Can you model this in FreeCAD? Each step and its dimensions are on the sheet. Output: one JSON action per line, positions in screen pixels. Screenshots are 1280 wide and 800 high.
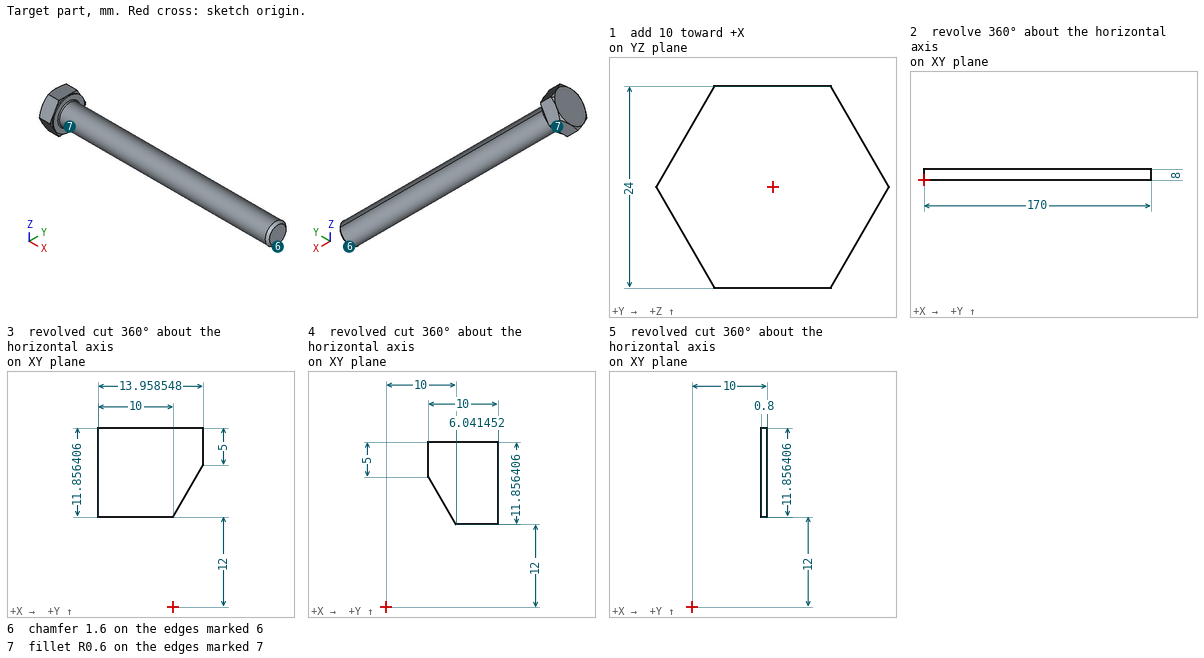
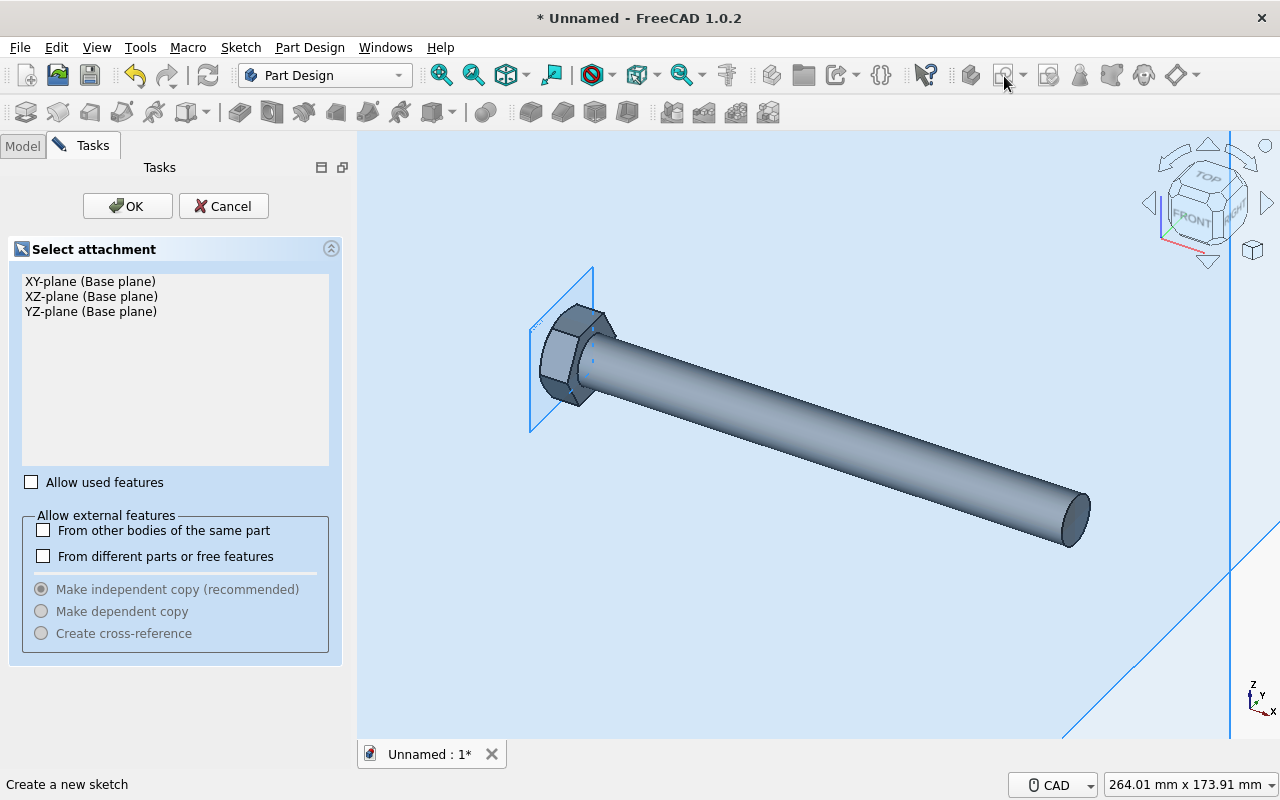
{"action": "left_click", "coordinate": [82, 282]}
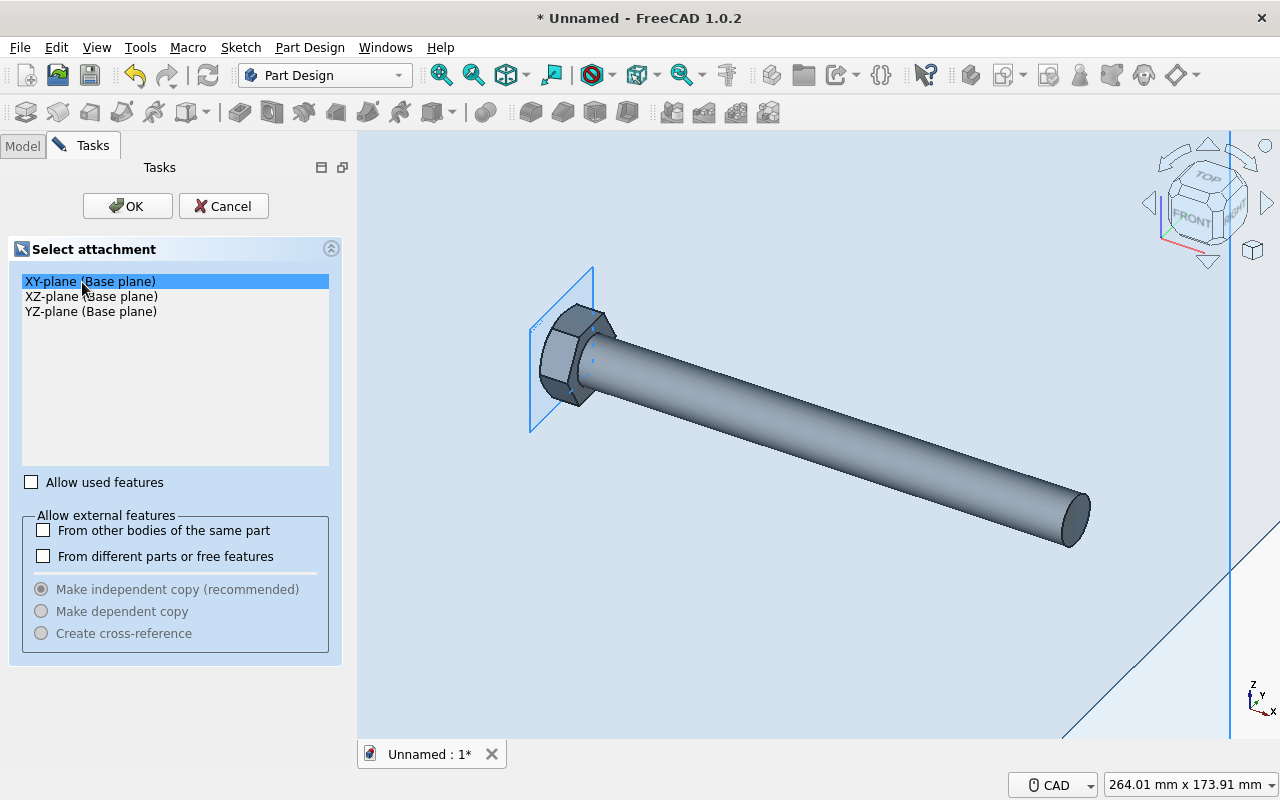
{"action": "left_click", "coordinate": [128, 206]}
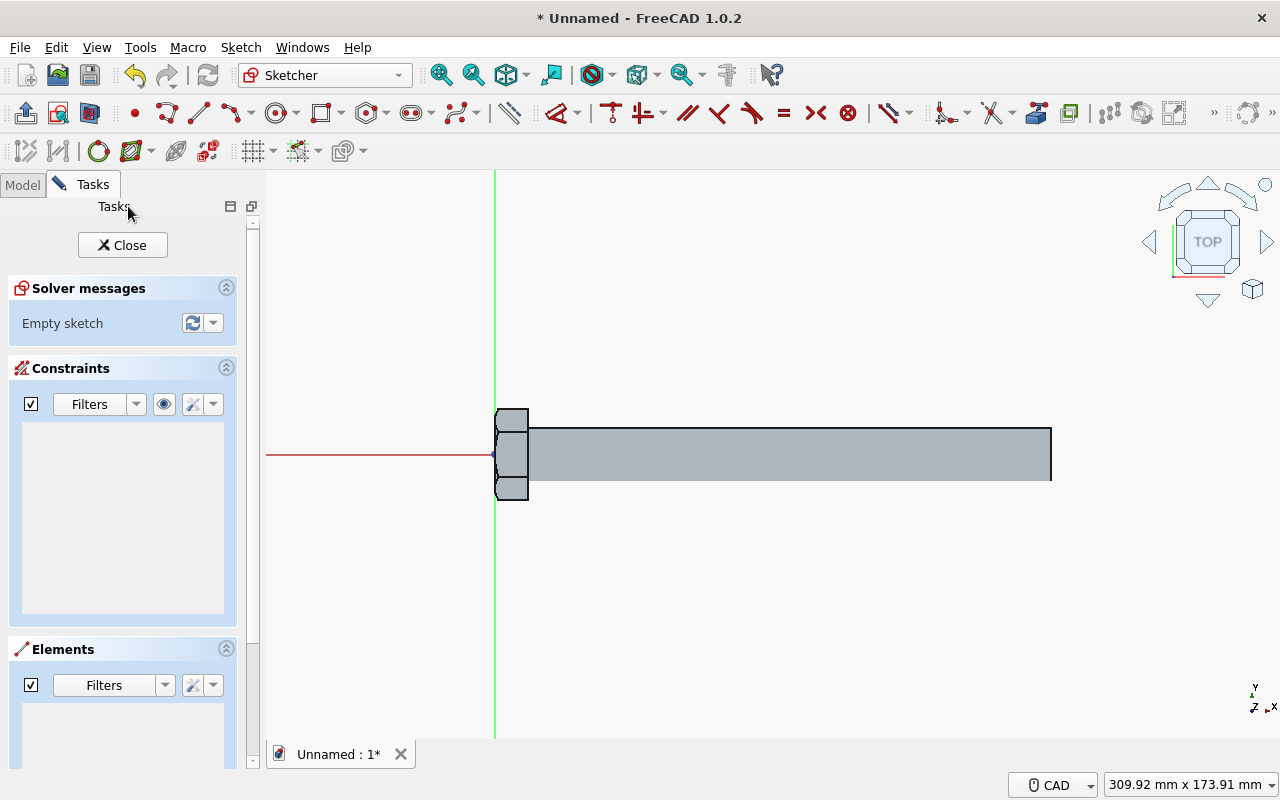
{"action": "left_click", "coordinate": [90, 114]}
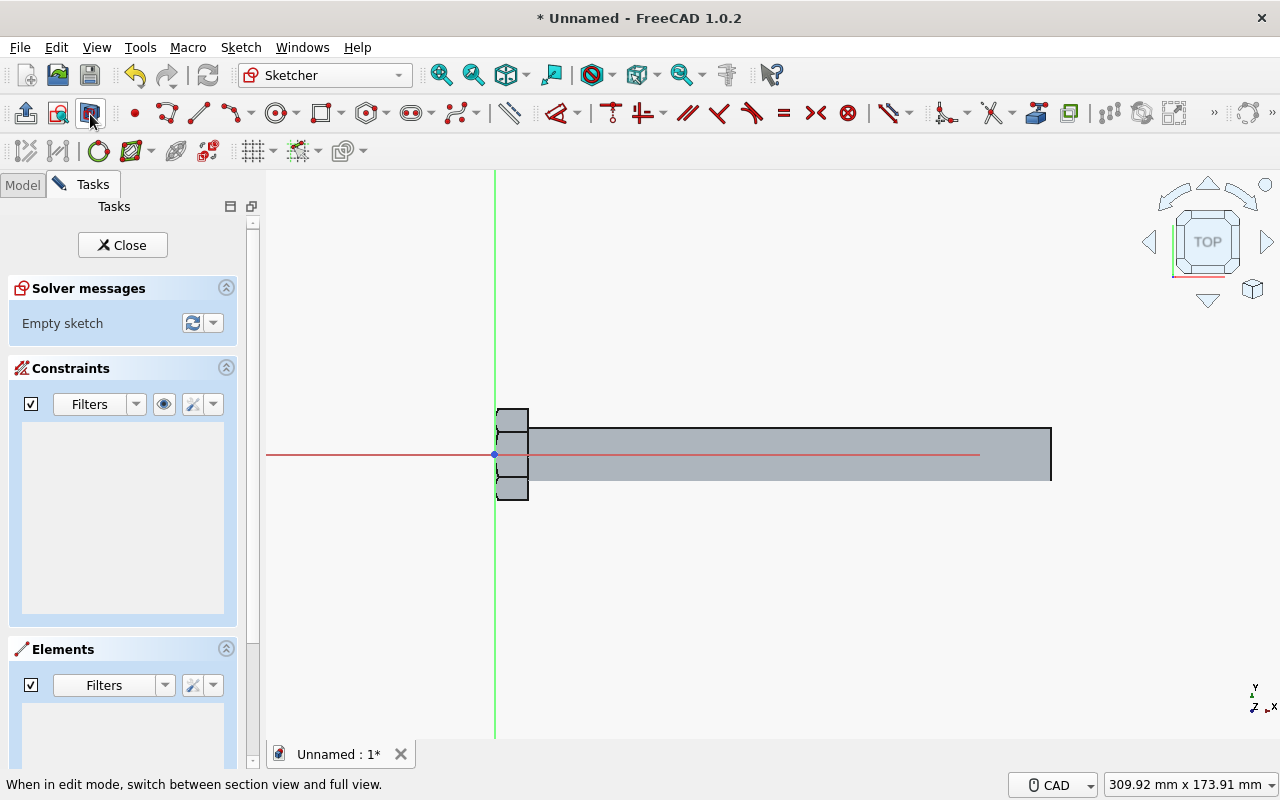
{"action": "scroll", "coordinate": [475, 406], "scroll_direction": "up", "scroll_amount": 8}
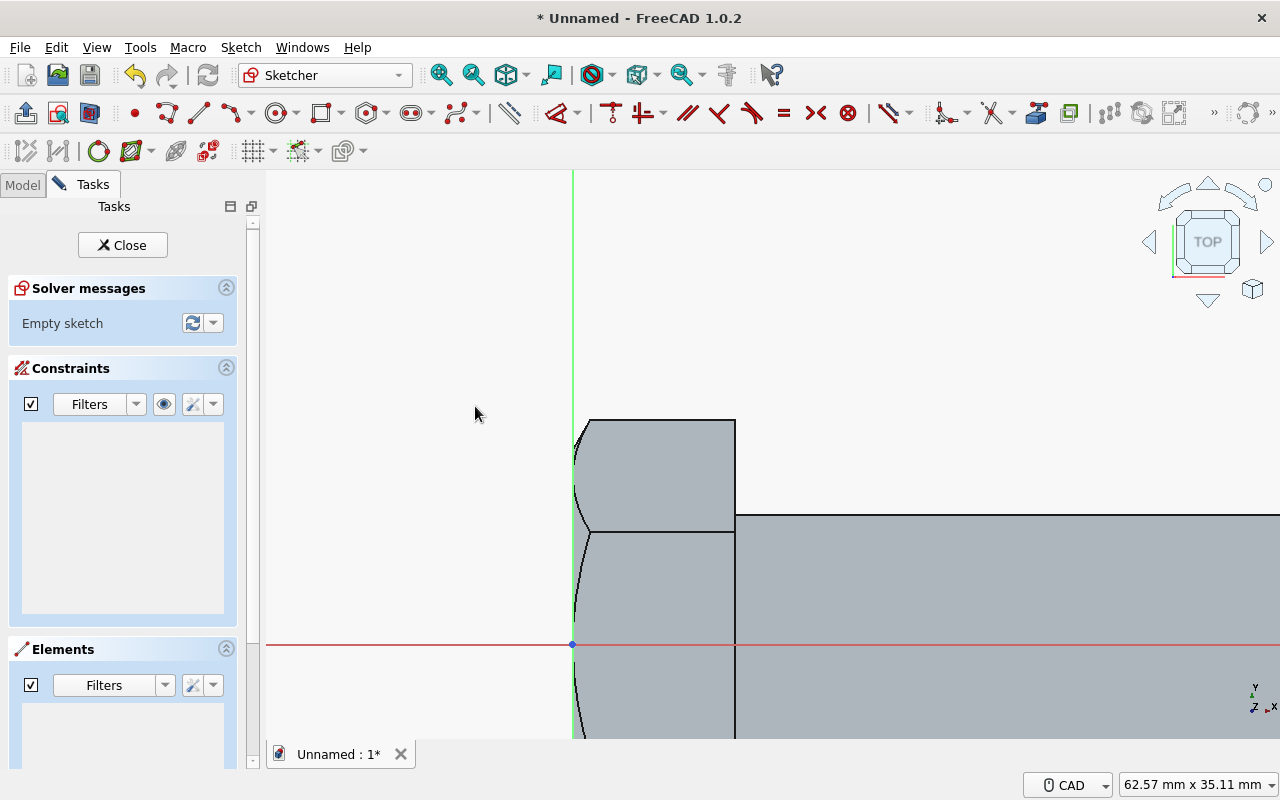
{"action": "left_click", "coordinate": [168, 114]}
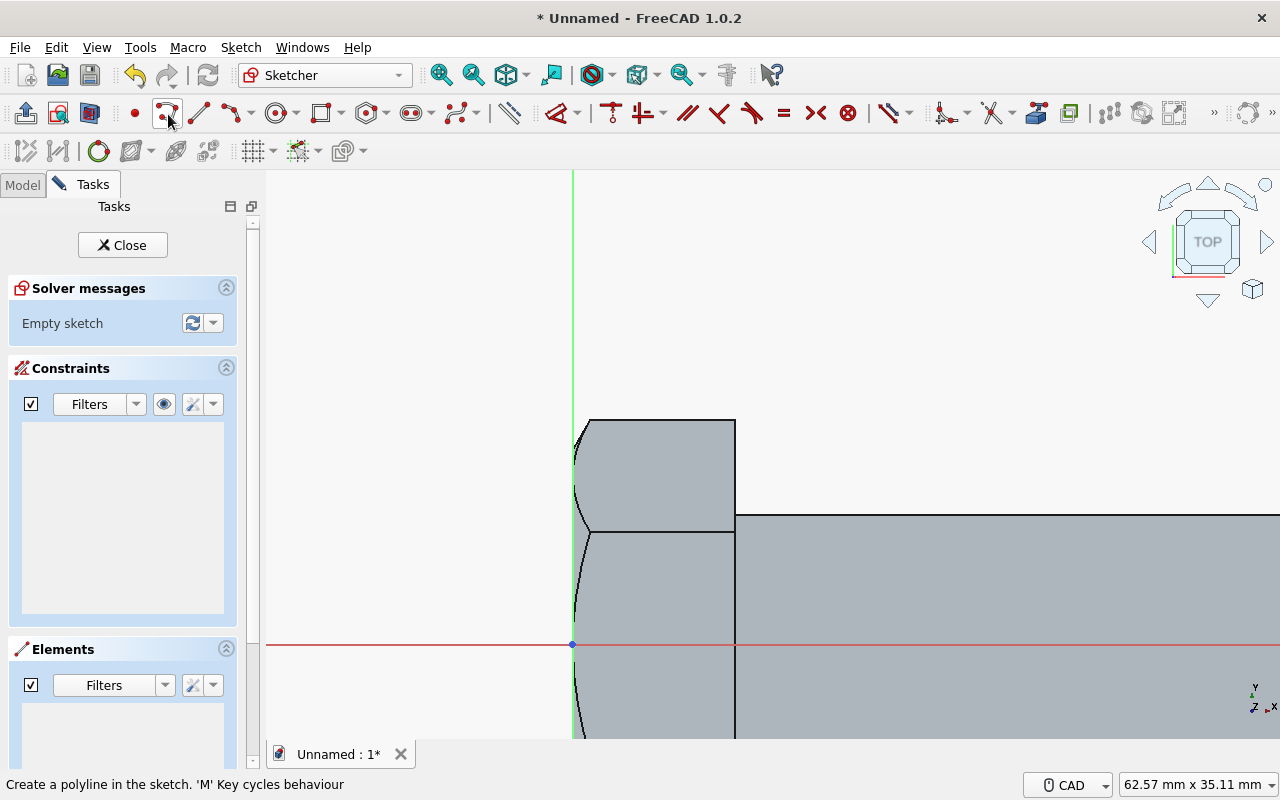
{"action": "left_click", "coordinate": [735, 450]}
{"action": "left_click", "coordinate": [833, 450]}
{"action": "left_click", "coordinate": [833, 258]}
{"action": "left_click", "coordinate": [671, 258]}
{"action": "left_click", "coordinate": [671, 339]}
{"action": "left_click", "coordinate": [735, 451]}
{"action": "key", "text": "Escape"}
{"action": "key", "text": "Escape"}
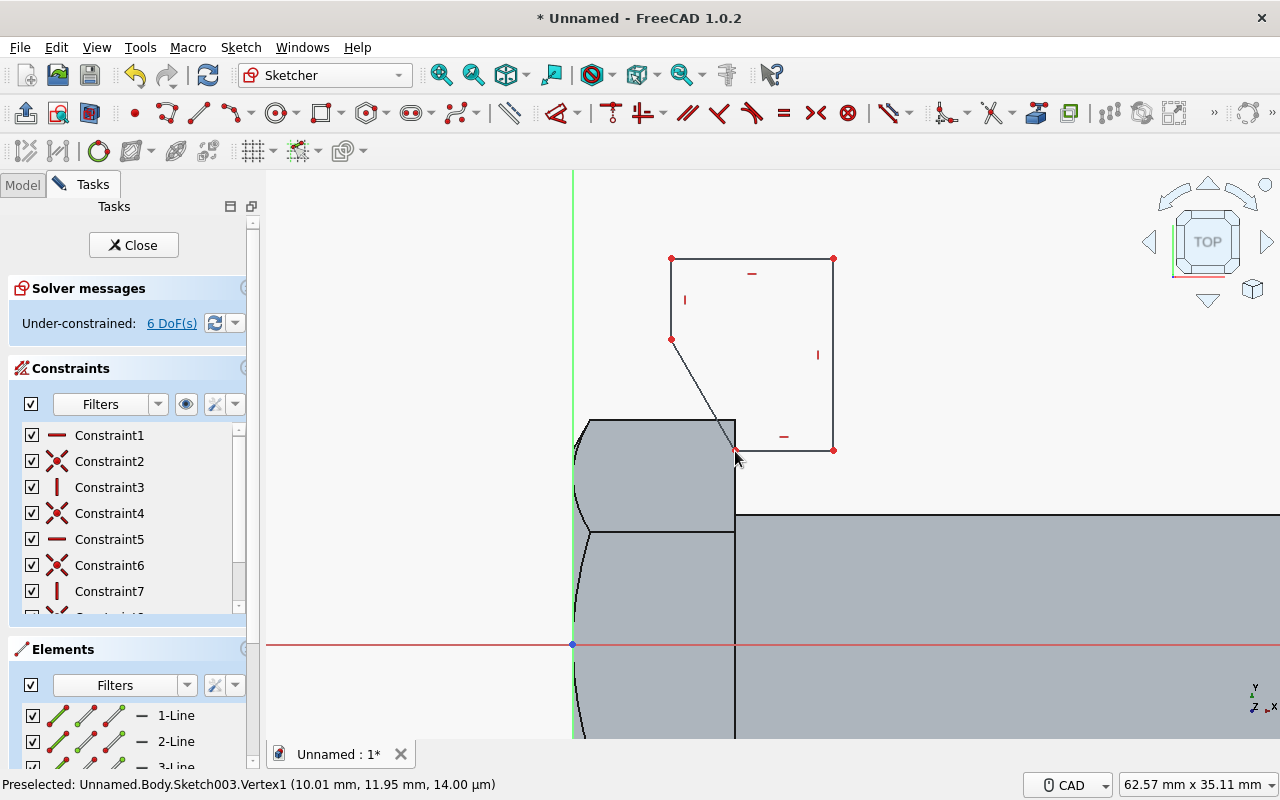
{"action": "left_click", "coordinate": [556, 114]}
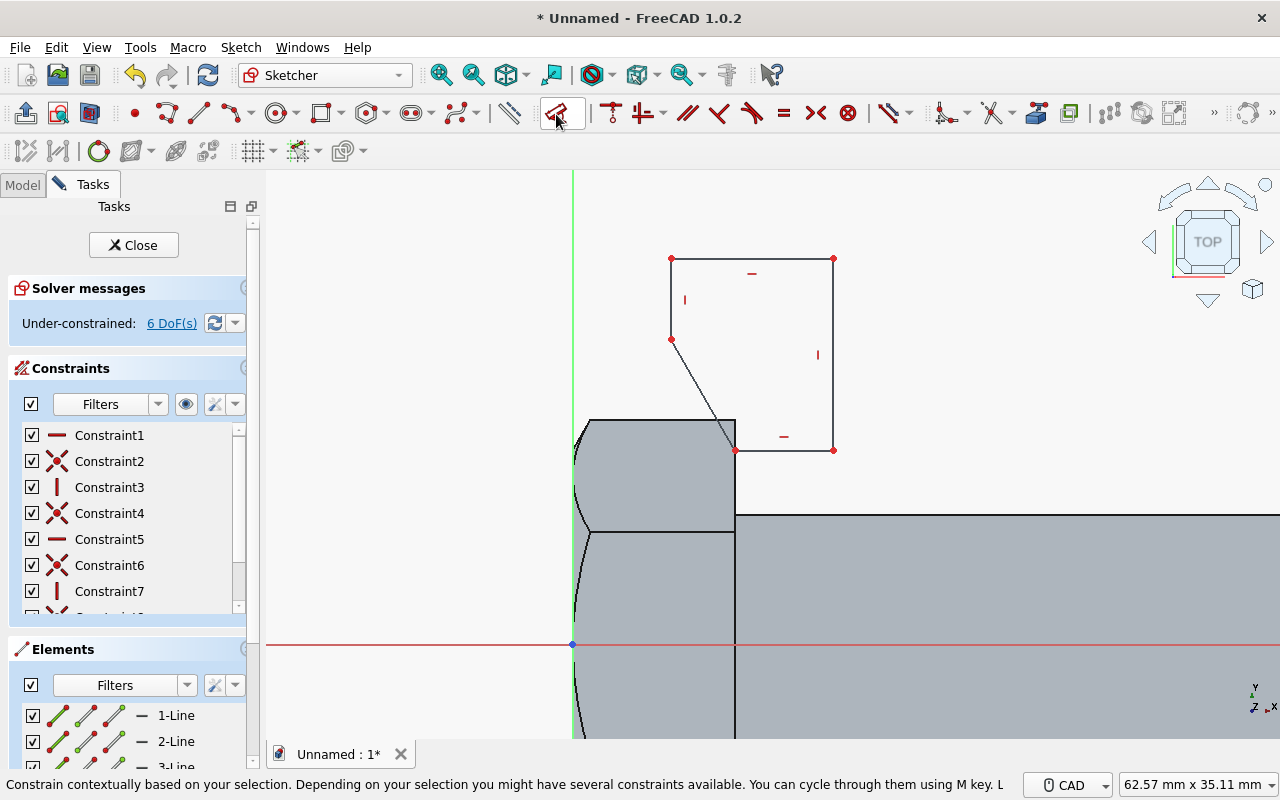
{"action": "left_click", "coordinate": [671, 283]}
{"action": "left_click", "coordinate": [637, 299]}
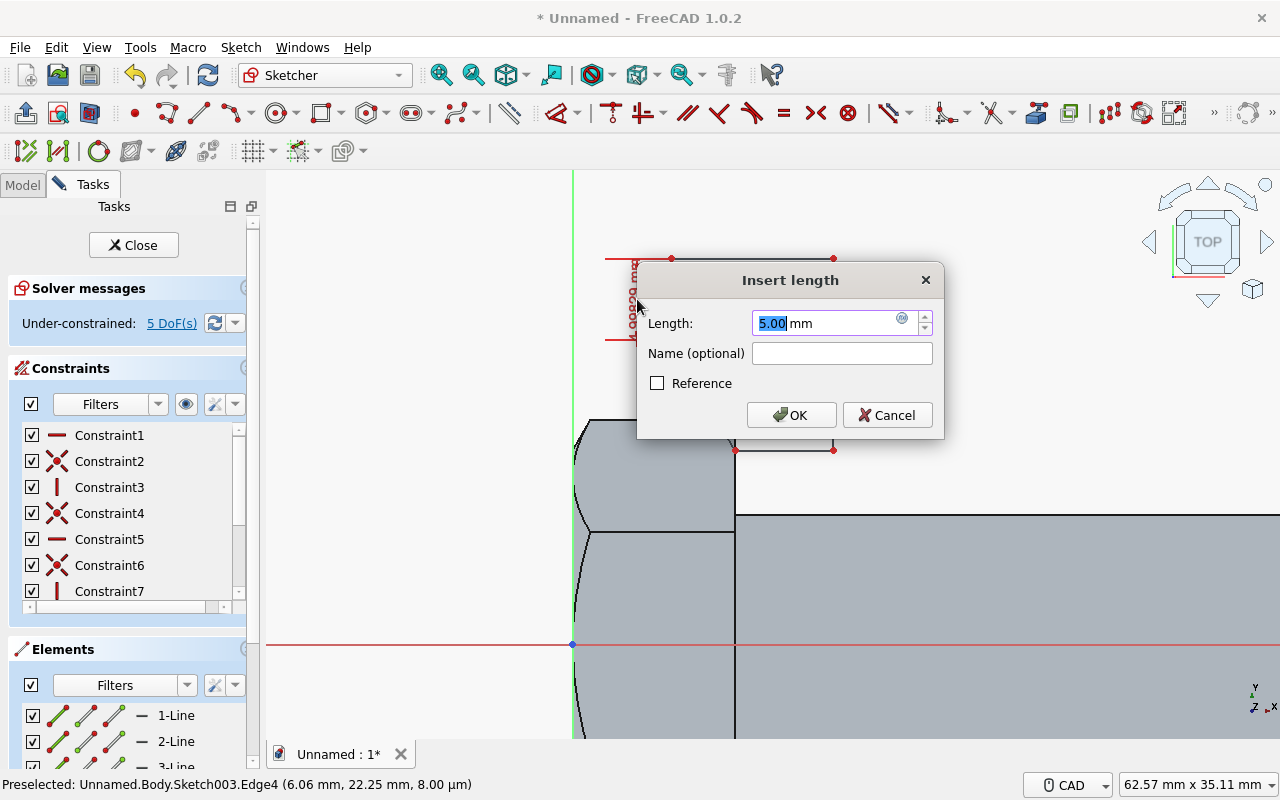
{"action": "type", "text": "5"}
{"action": "key", "text": "Return"}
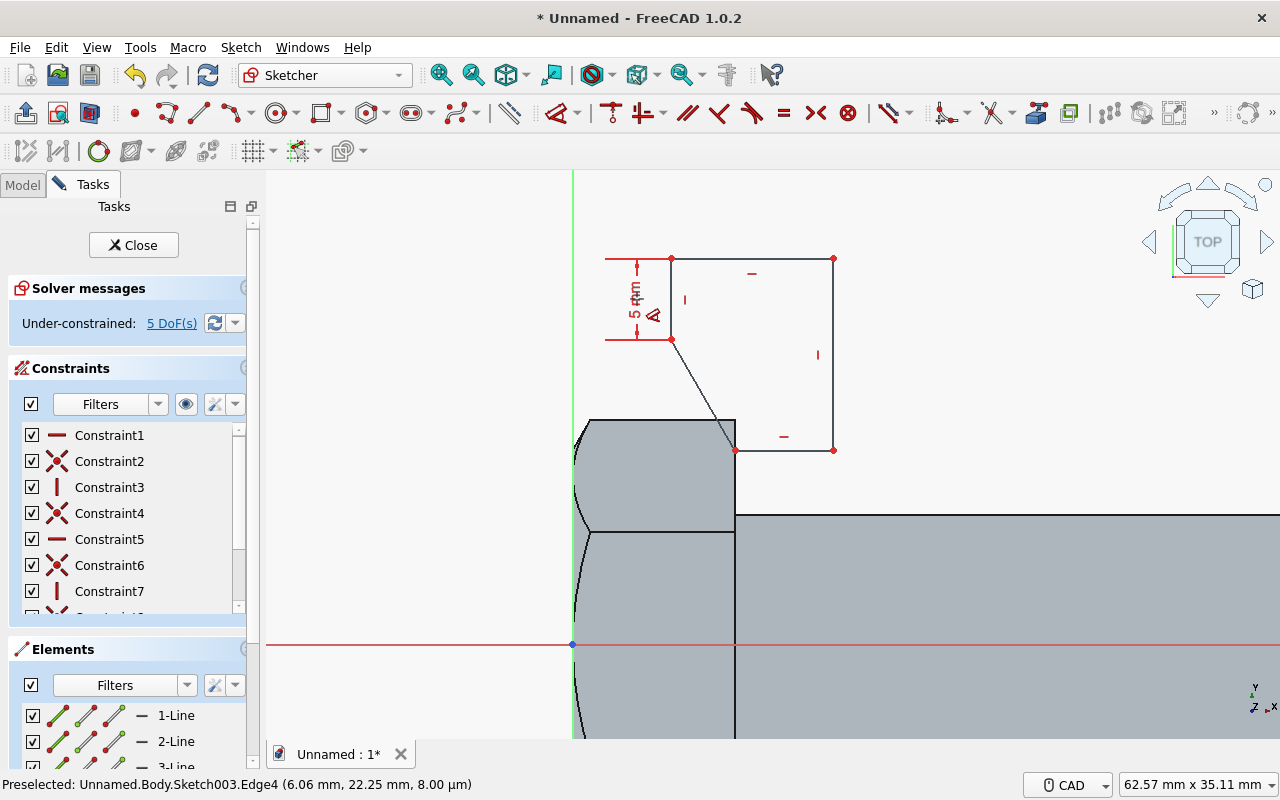
{"action": "left_click", "coordinate": [784, 259]}
{"action": "left_click", "coordinate": [752, 225]}